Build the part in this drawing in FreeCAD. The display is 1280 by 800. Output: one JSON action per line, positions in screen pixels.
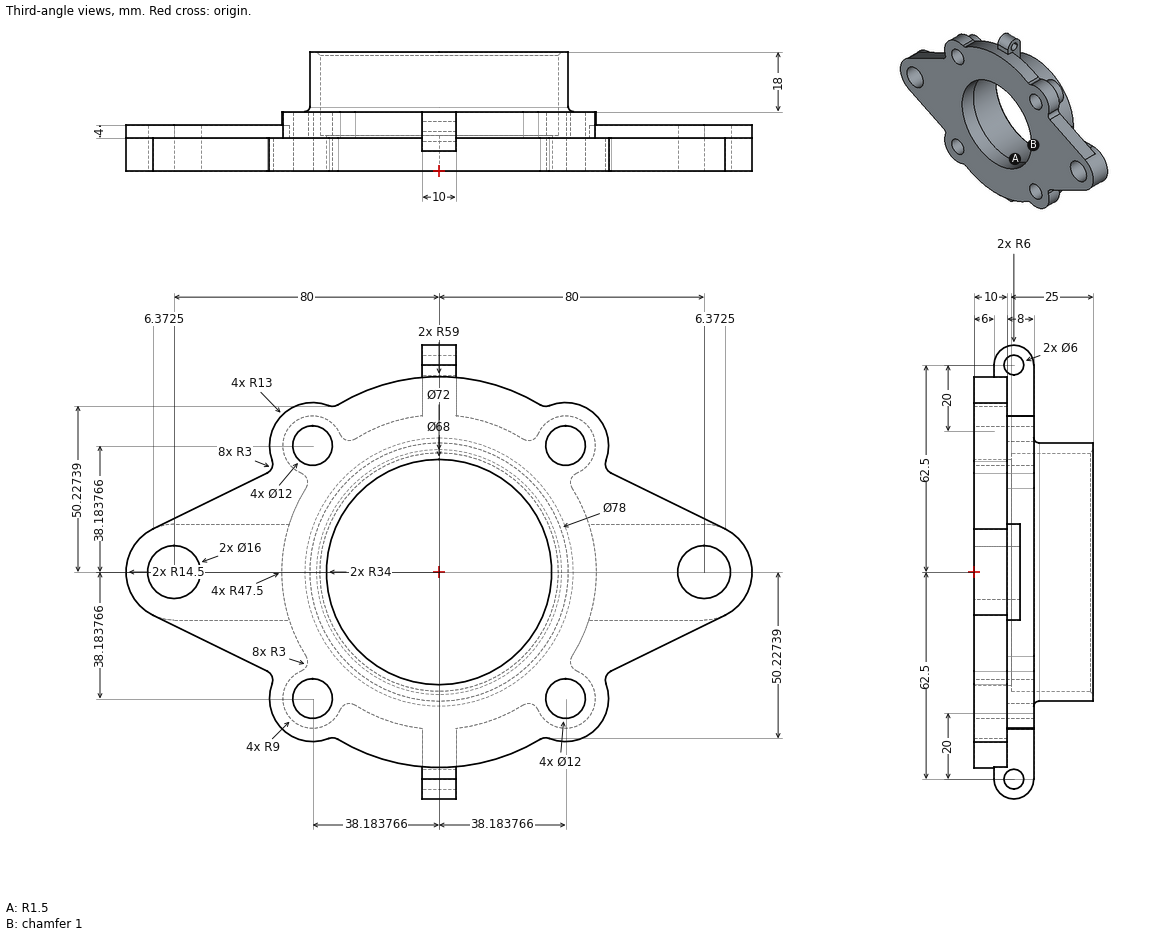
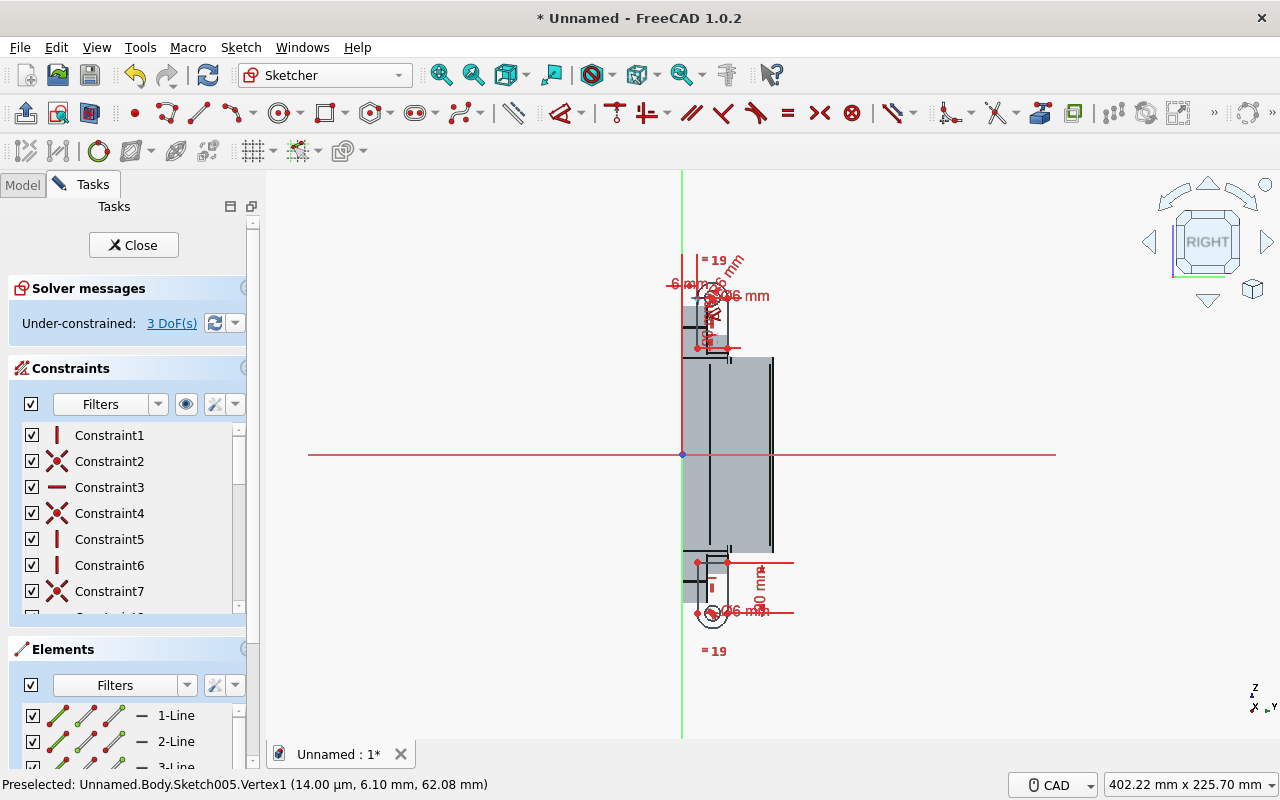
{"action": "scroll", "coordinate": [698, 563], "scroll_direction": "up", "scroll_amount": 5}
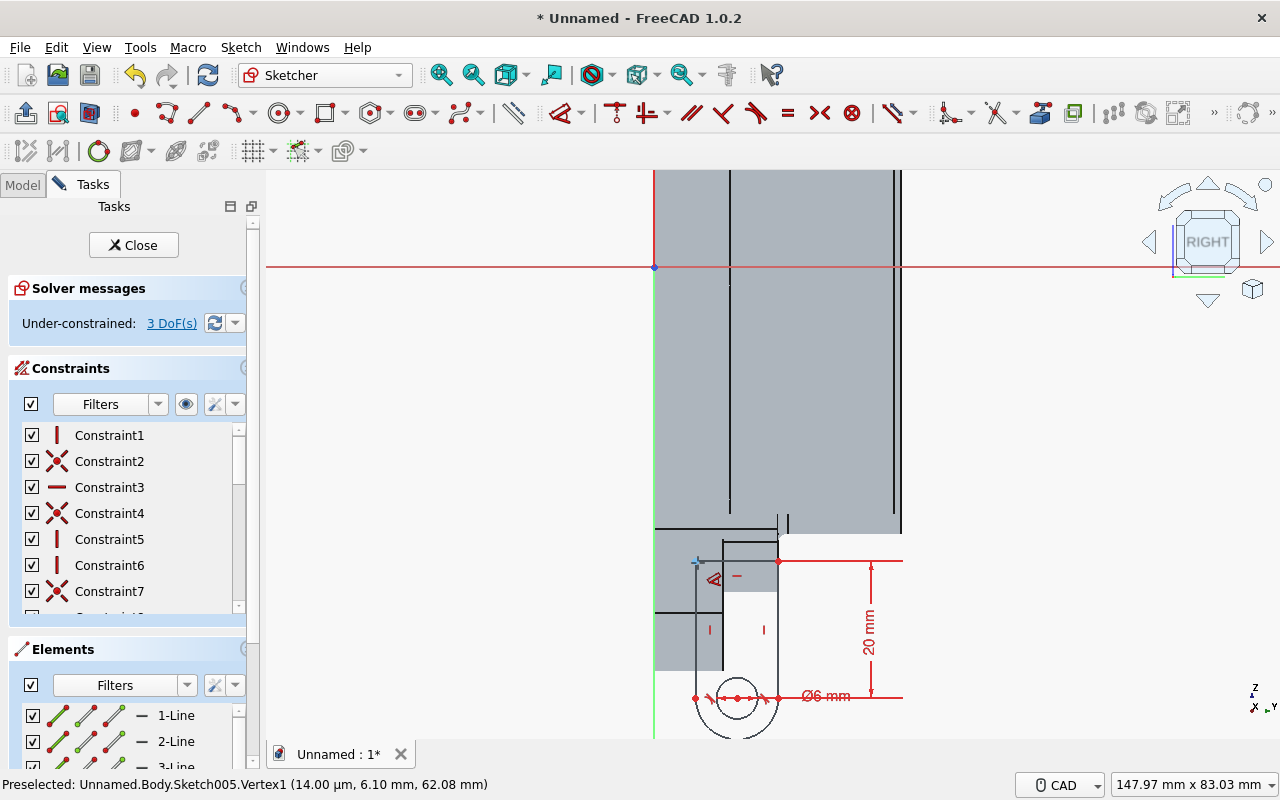
{"action": "left_click", "coordinate": [696, 561]}
{"action": "left_click", "coordinate": [675, 595]}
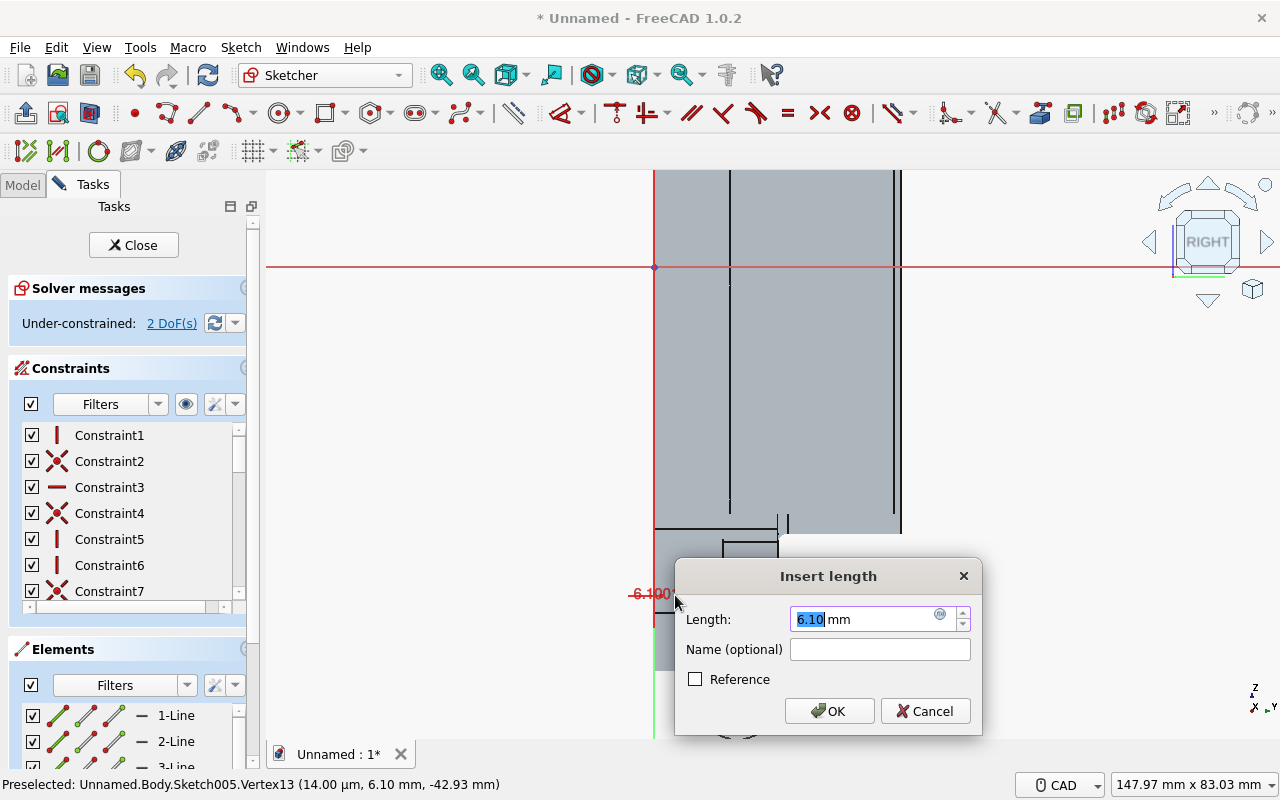
{"action": "type", "text": "6"}
{"action": "key", "text": "Return"}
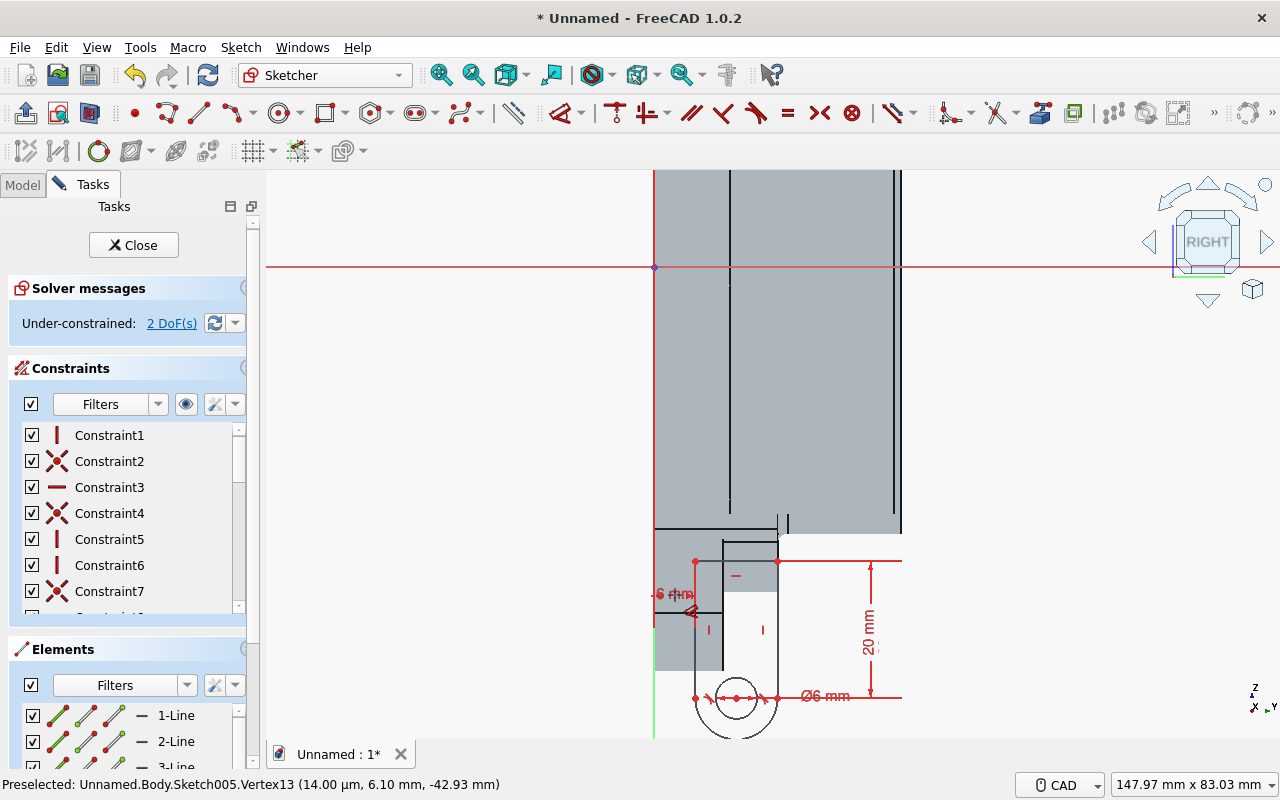
{"action": "scroll", "coordinate": [698, 564], "scroll_direction": "down", "scroll_amount": 5}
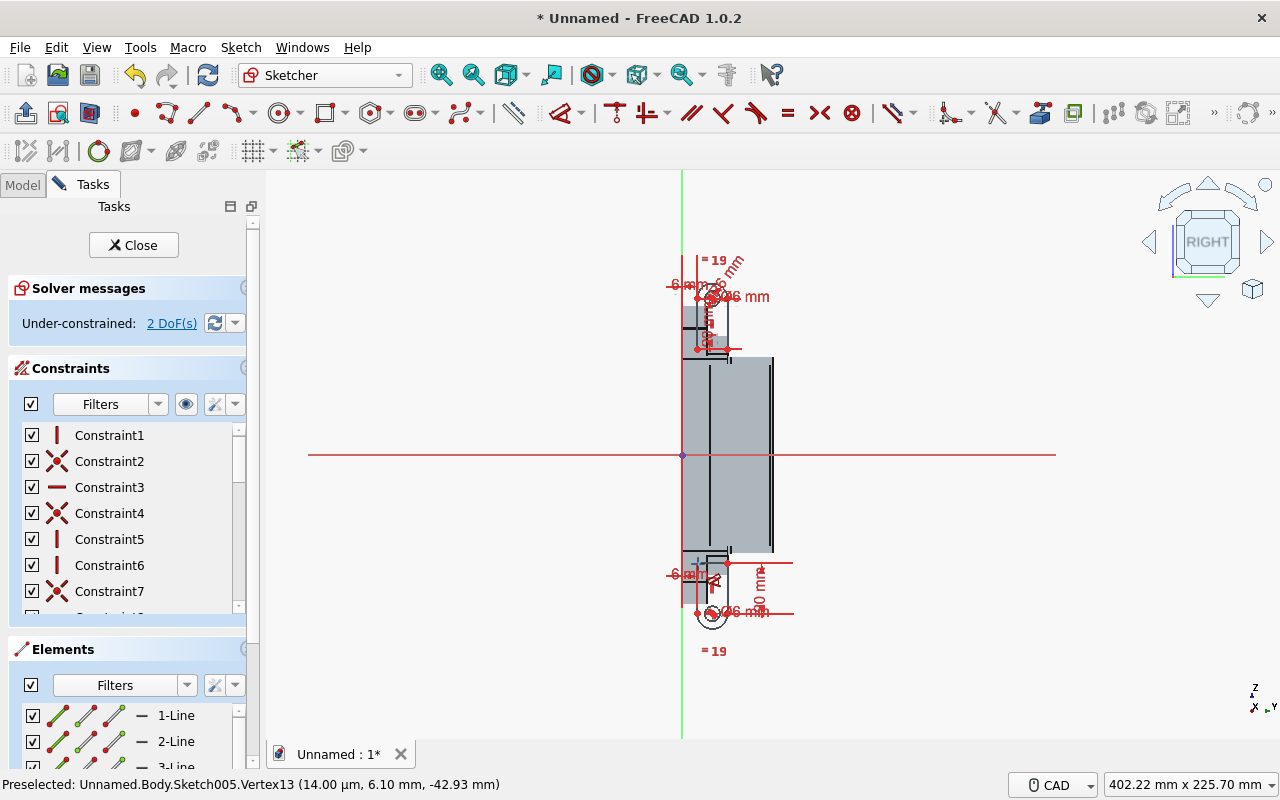
{"action": "left_click", "coordinate": [712, 299]}
{"action": "left_click", "coordinate": [648, 377]}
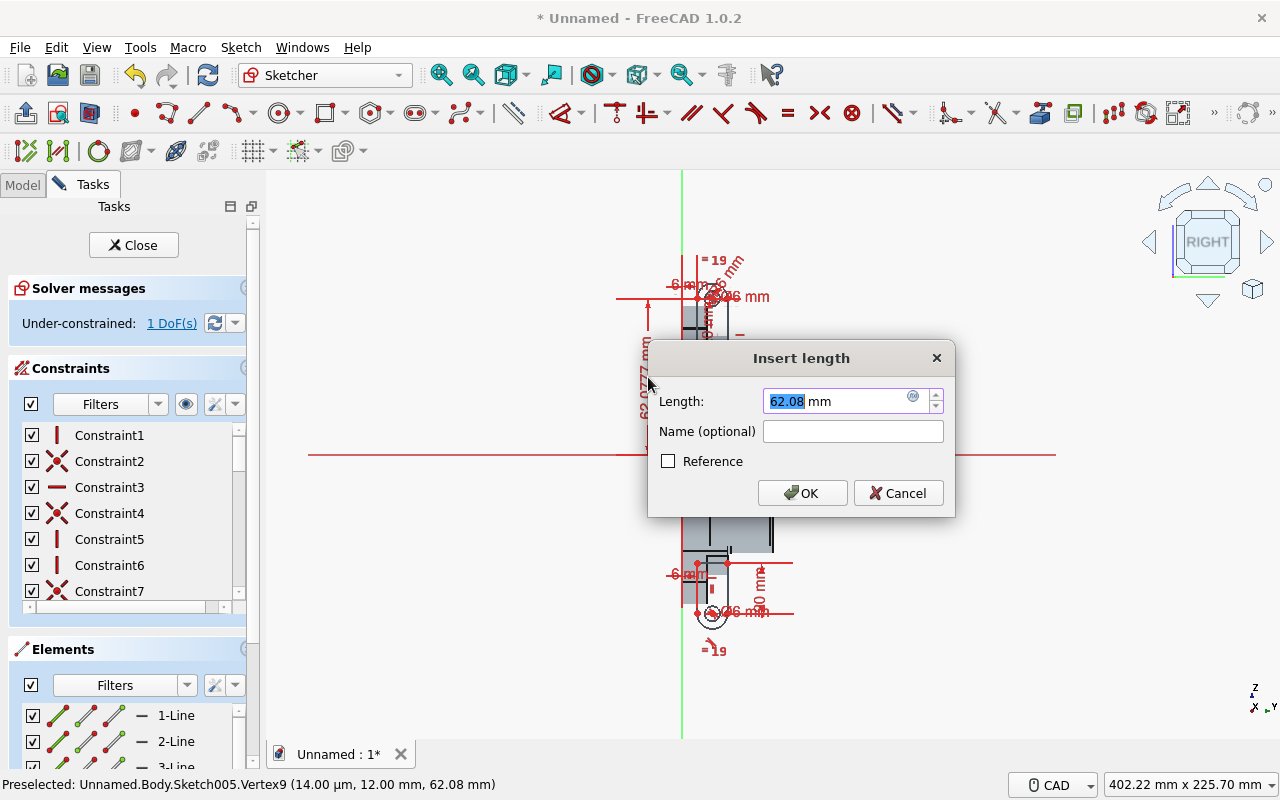
{"action": "type", "text": "62.5"}
{"action": "key", "text": "Return"}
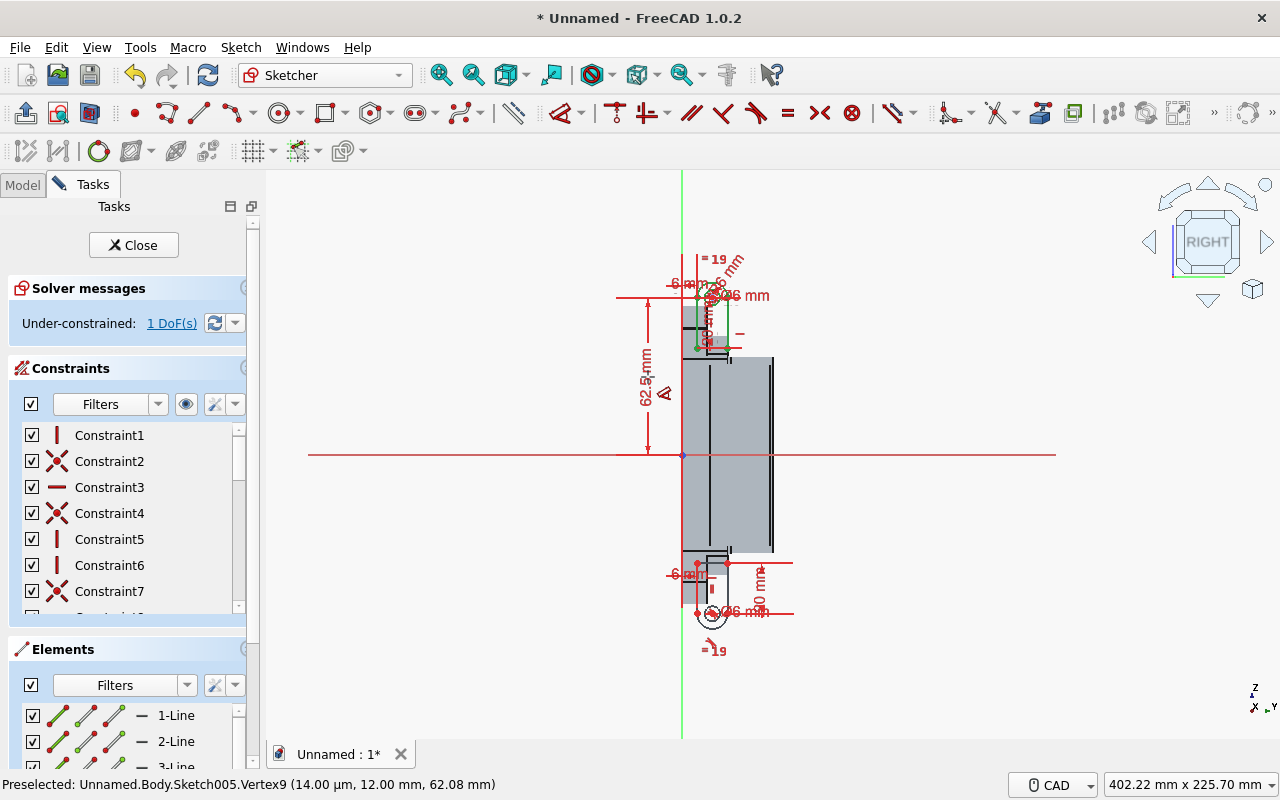
{"action": "left_click", "coordinate": [712, 614]}
{"action": "left_click", "coordinate": [648, 535]}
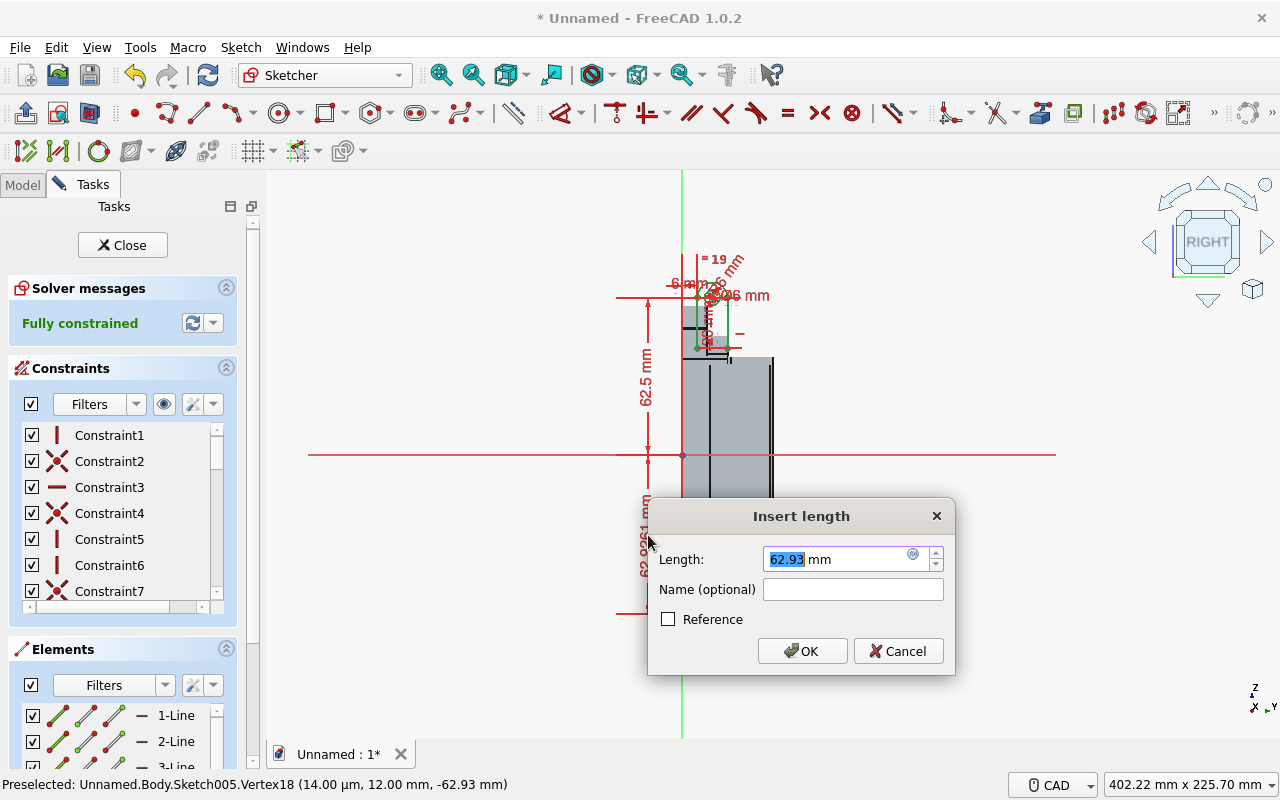
{"action": "type", "text": "62.5"}
{"action": "key", "text": "Return"}
{"action": "key", "text": "Escape"}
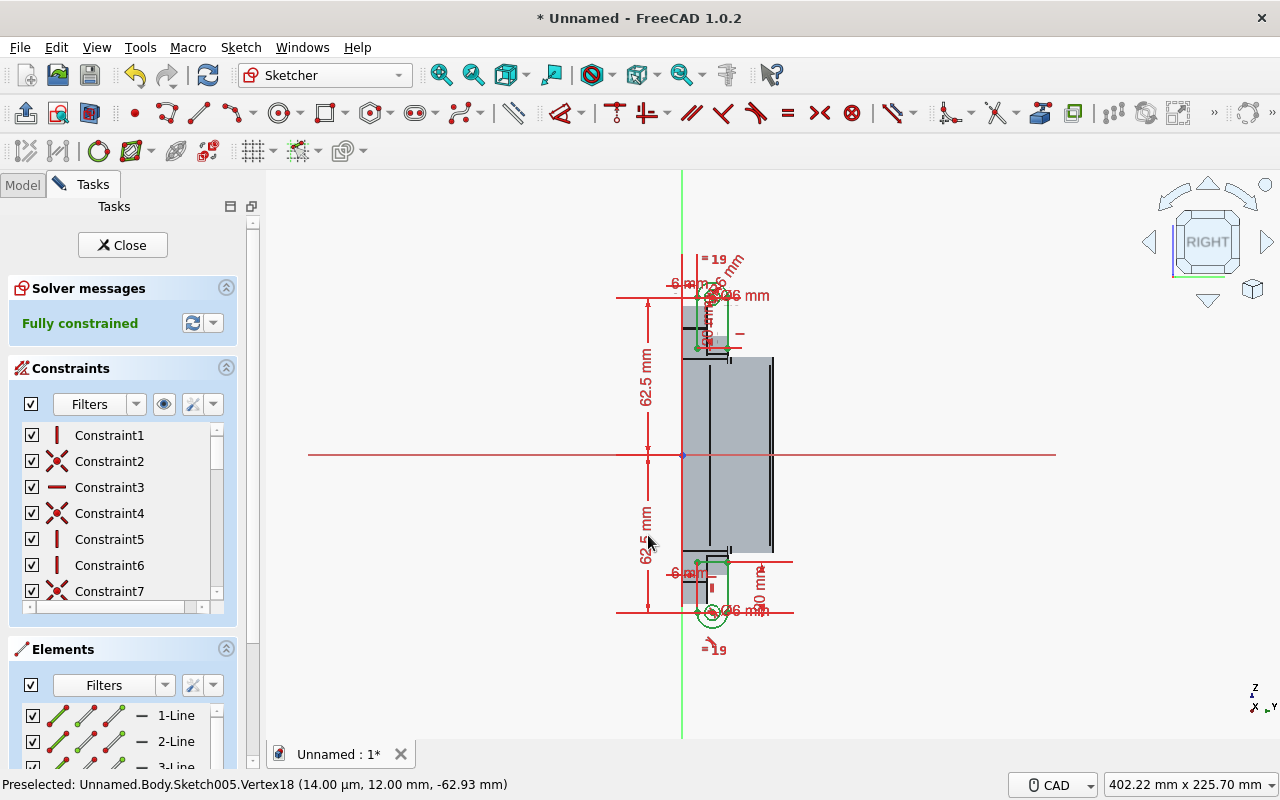
{"action": "left_click", "coordinate": [123, 245]}